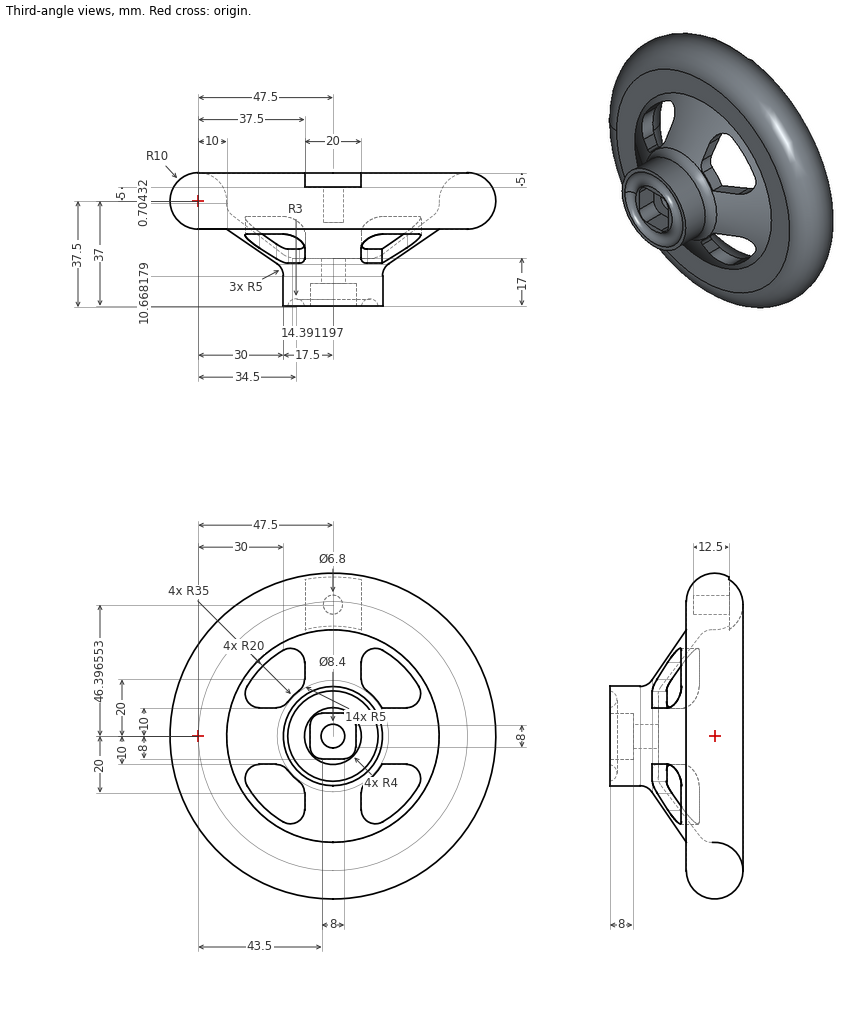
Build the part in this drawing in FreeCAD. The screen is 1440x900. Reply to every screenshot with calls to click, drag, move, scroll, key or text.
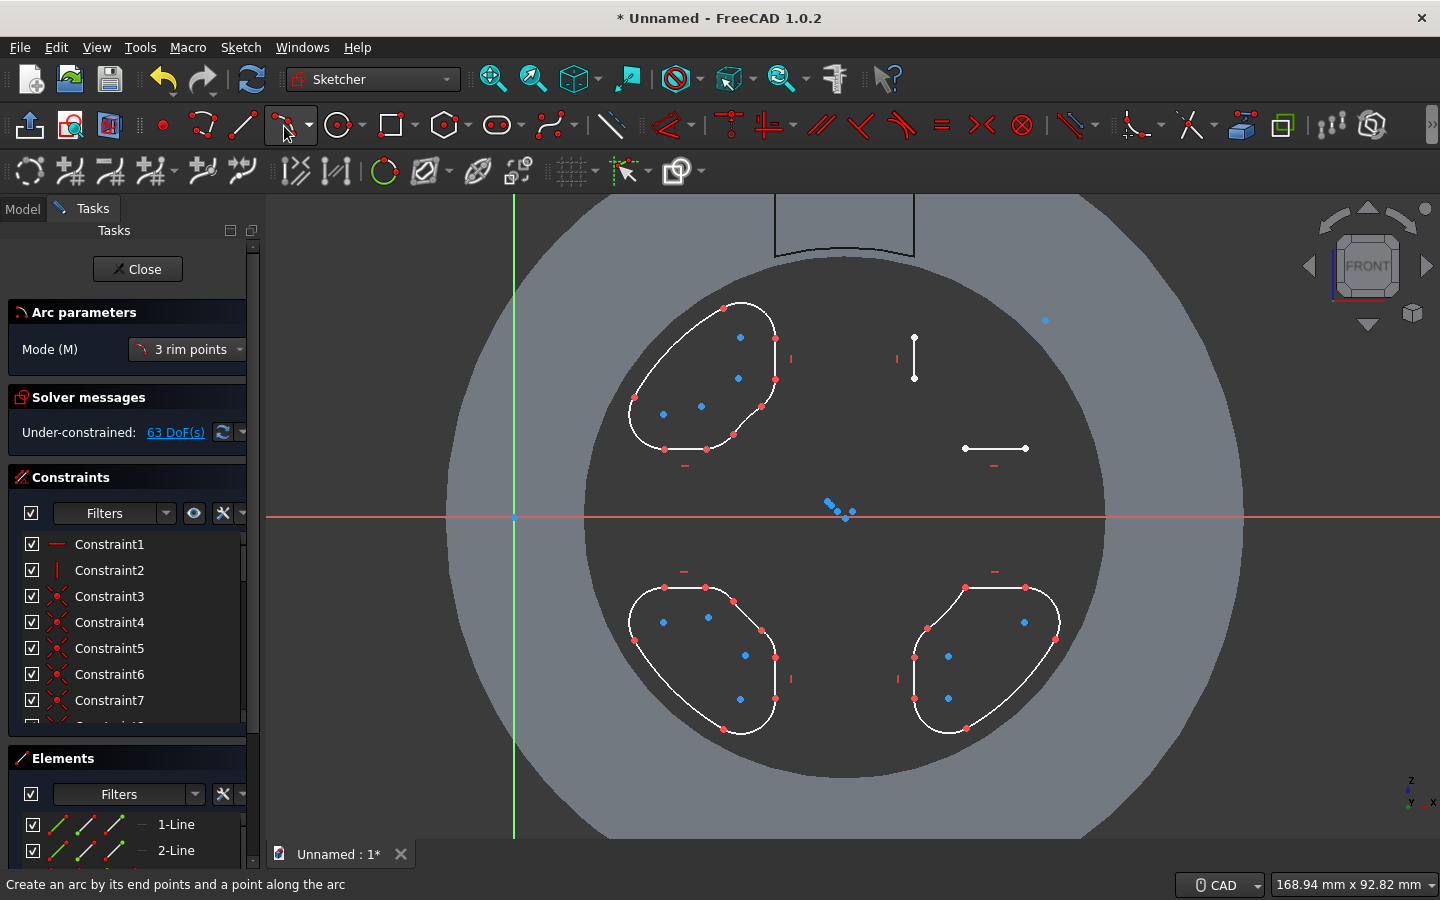
click(965, 449)
click(928, 406)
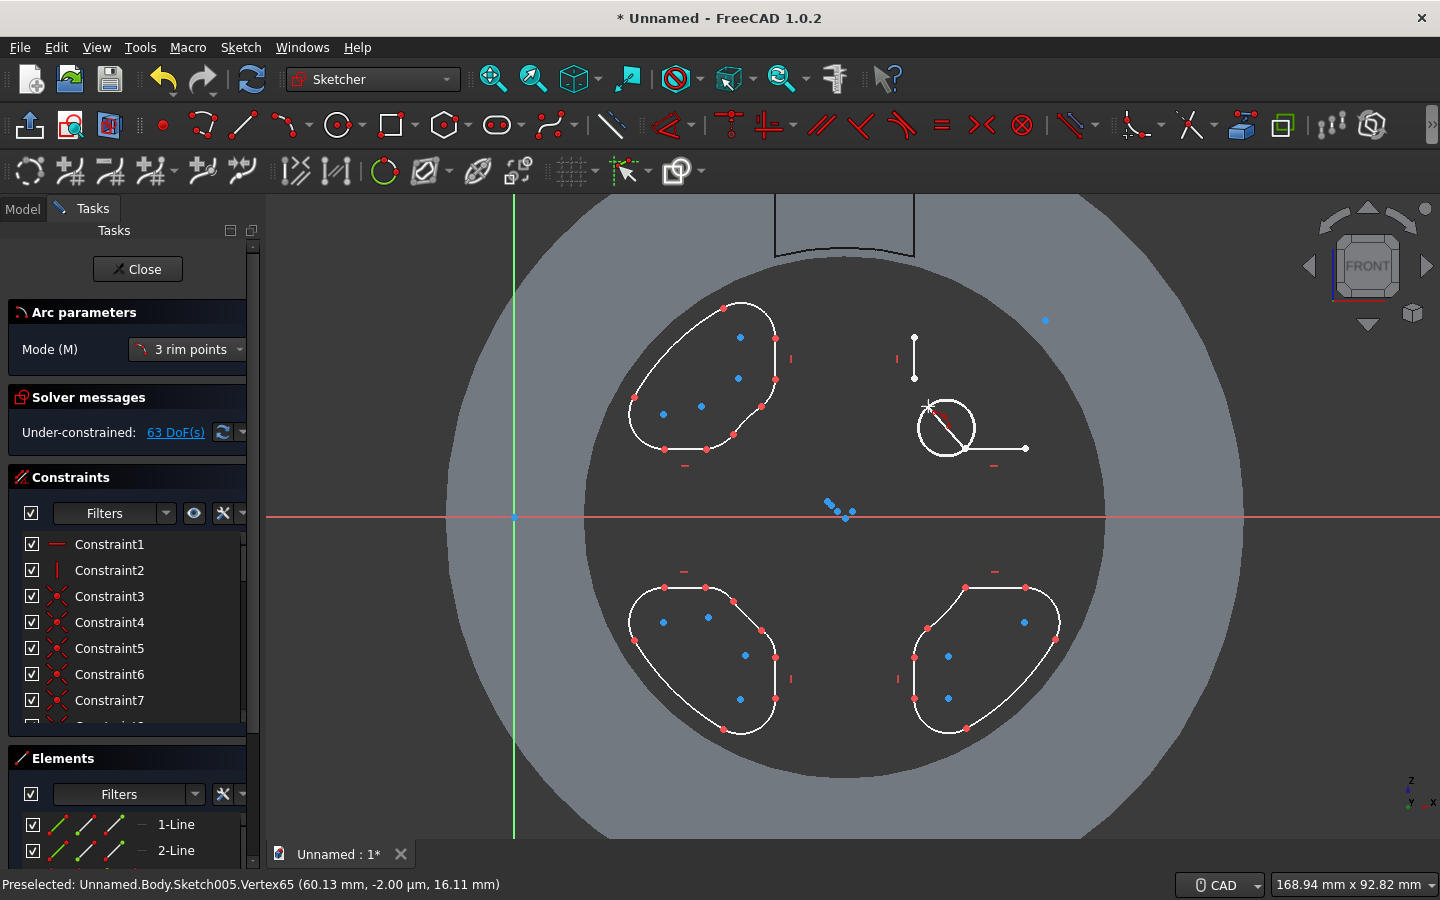
scroll(949, 425, up, 9)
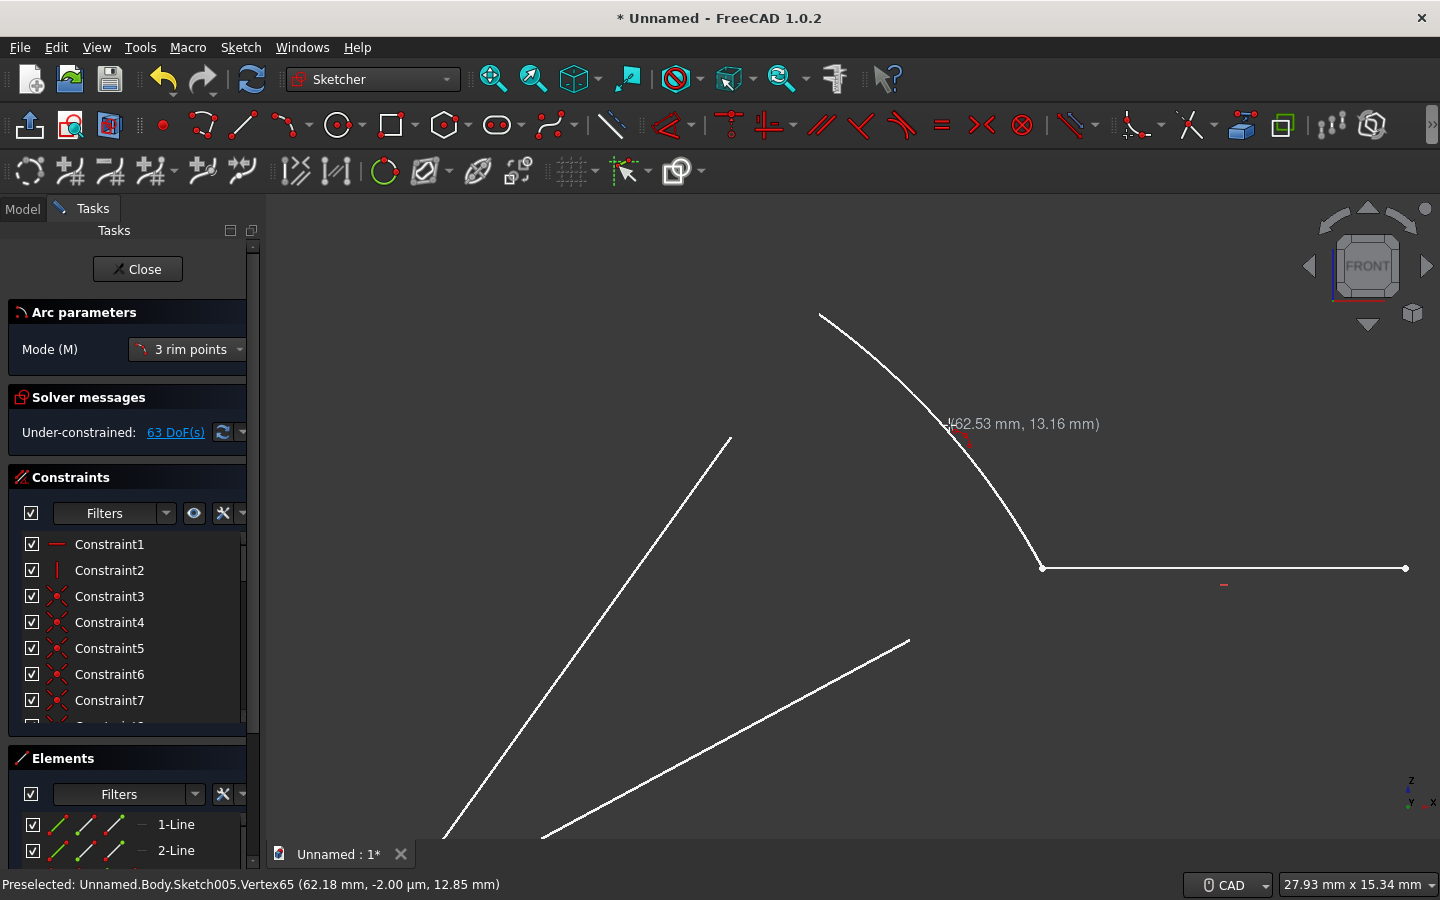
click(943, 425)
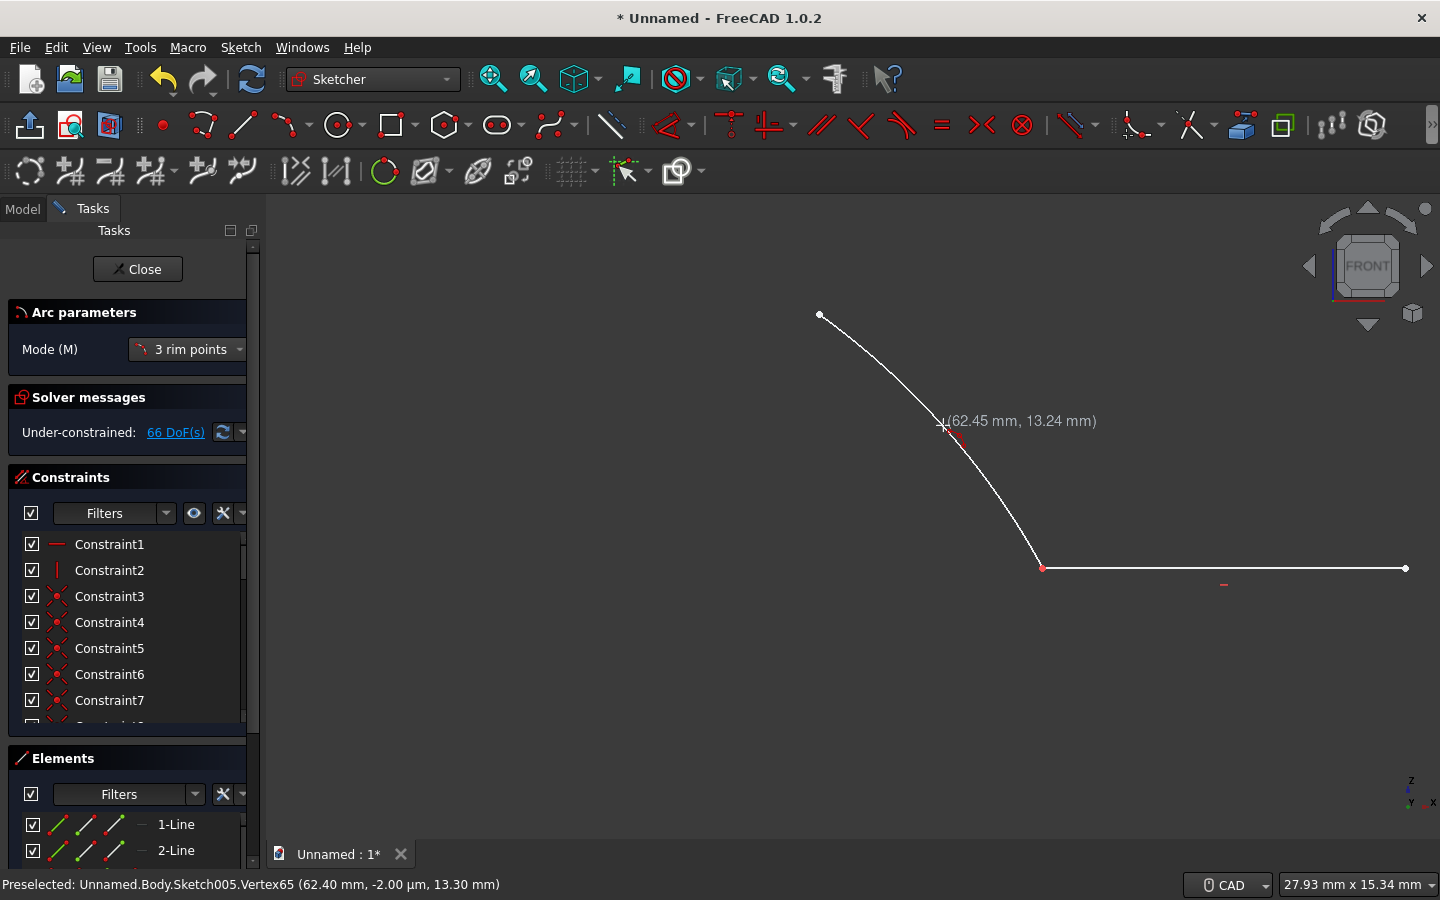
scroll(949, 424, down, 9)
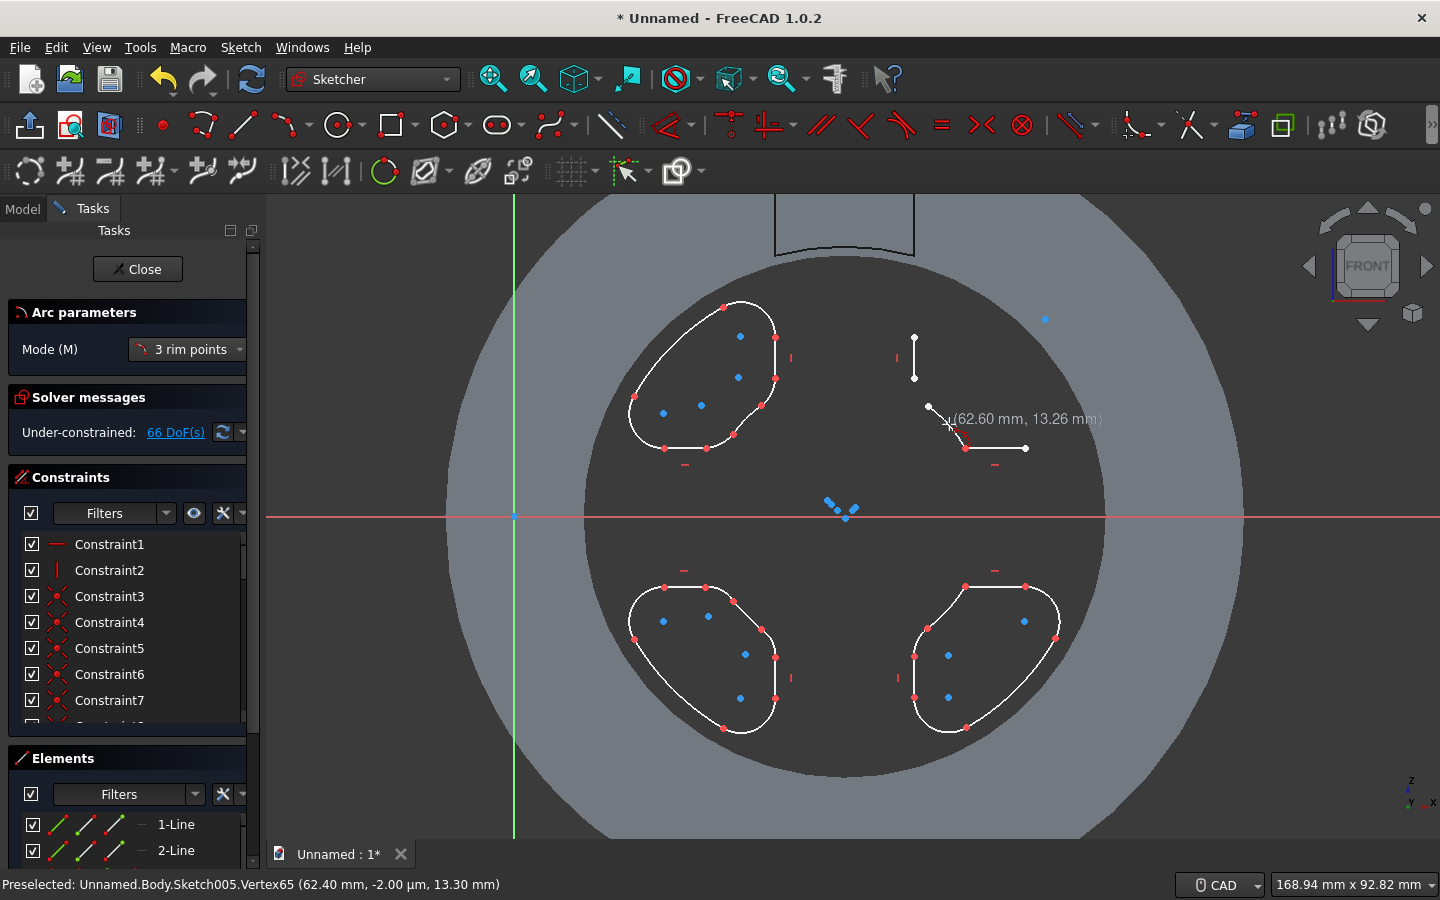
click(928, 406)
click(914, 378)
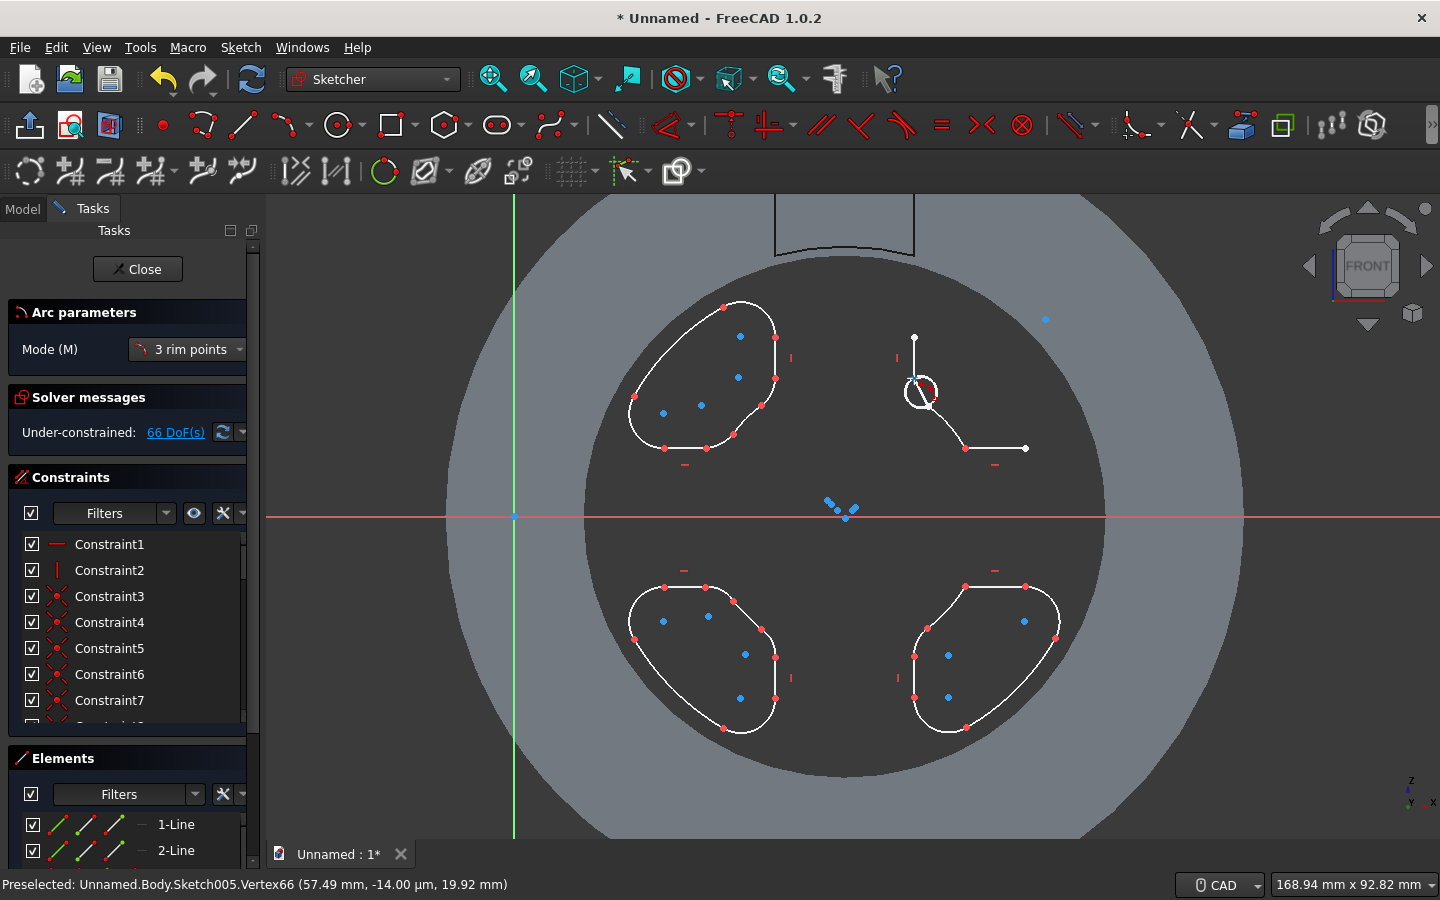
scroll(918, 393, up, 8)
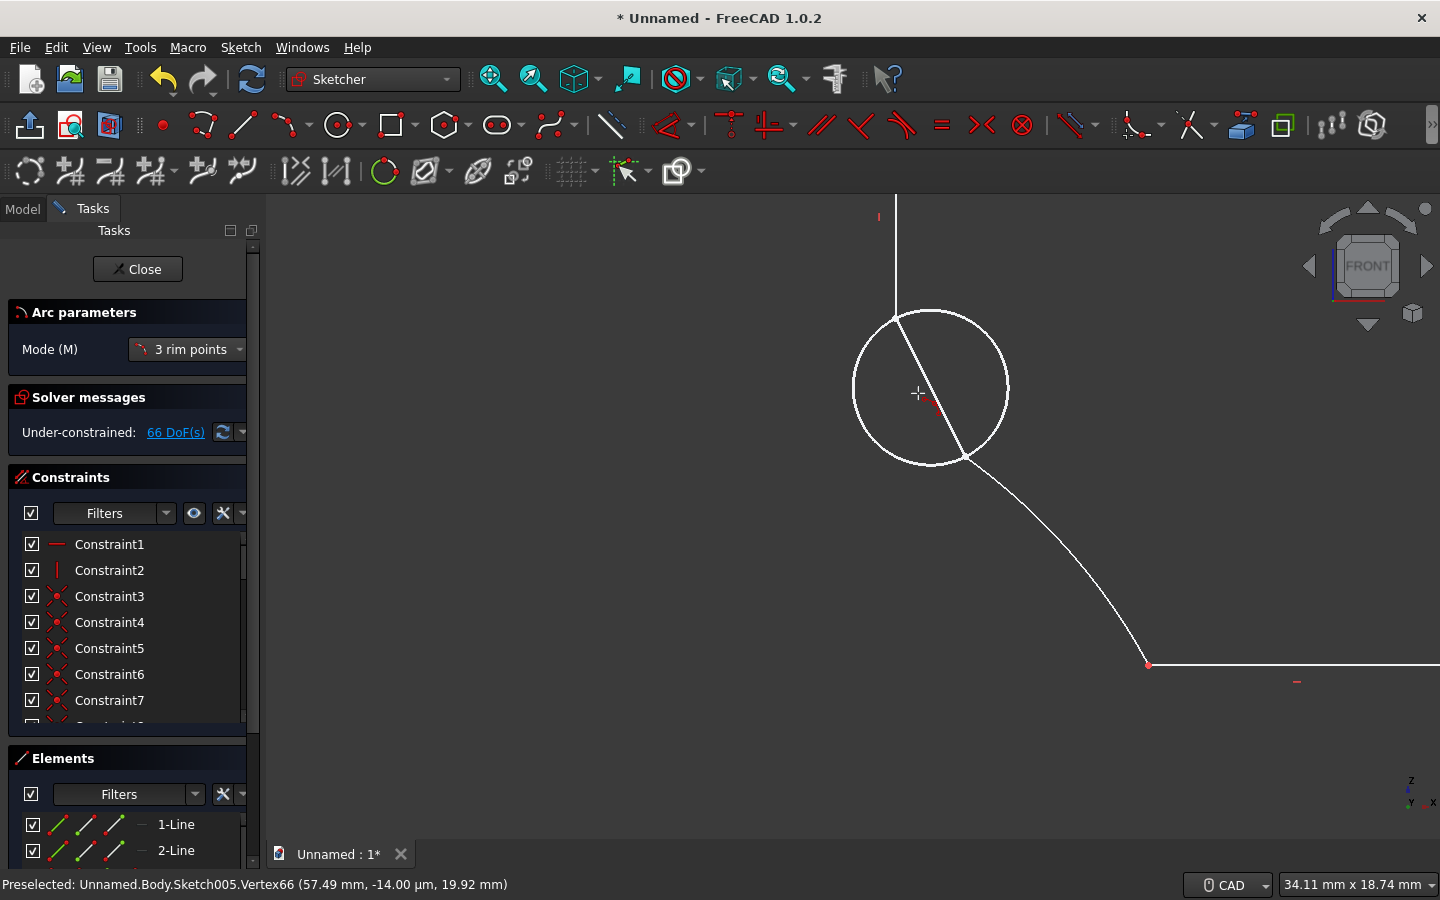
click(915, 393)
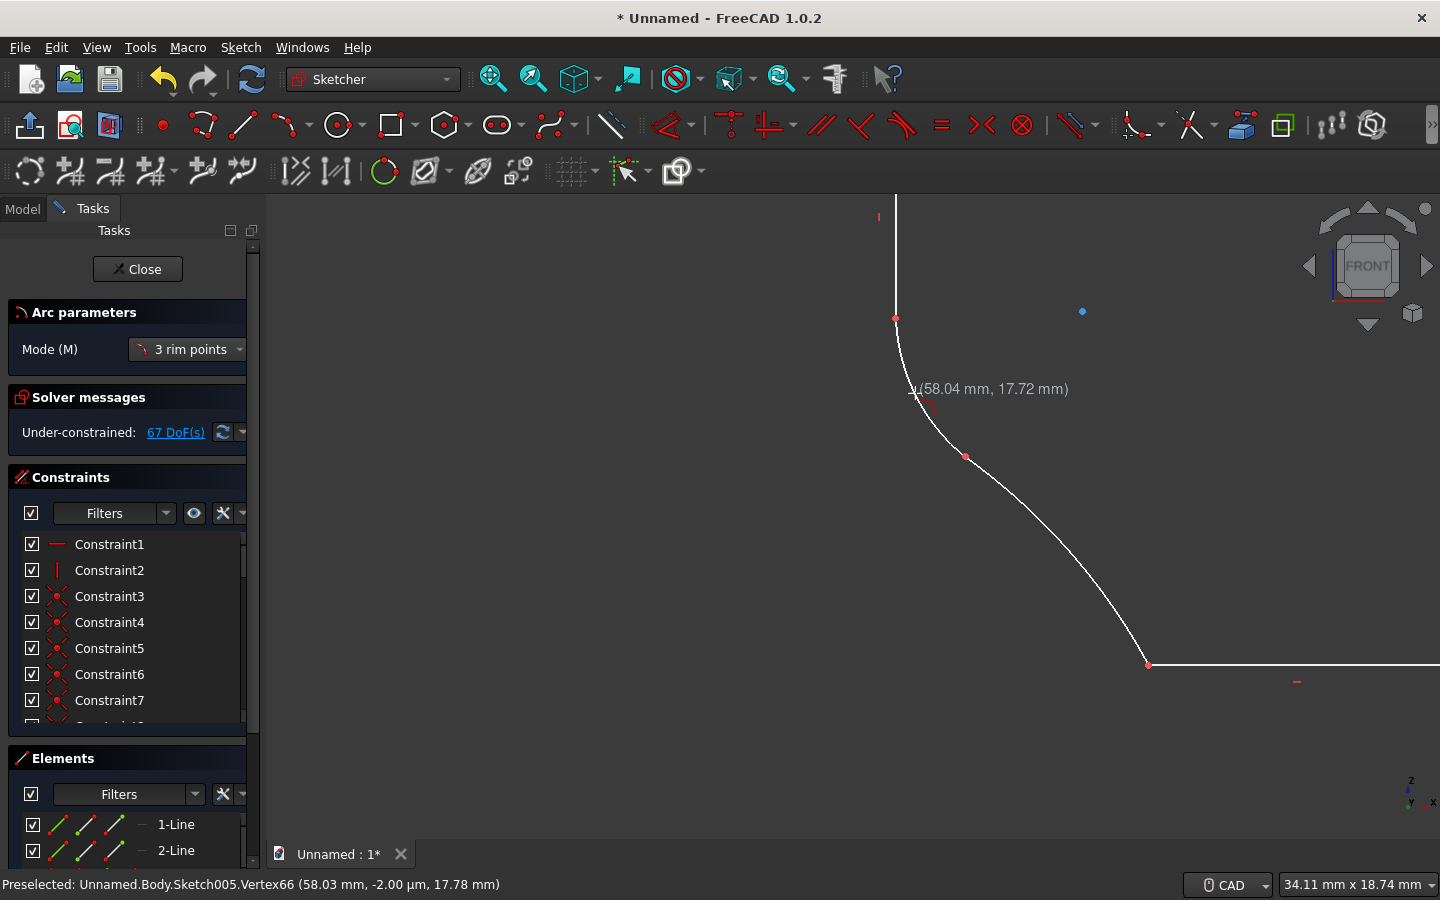
scroll(918, 393, down, 8)